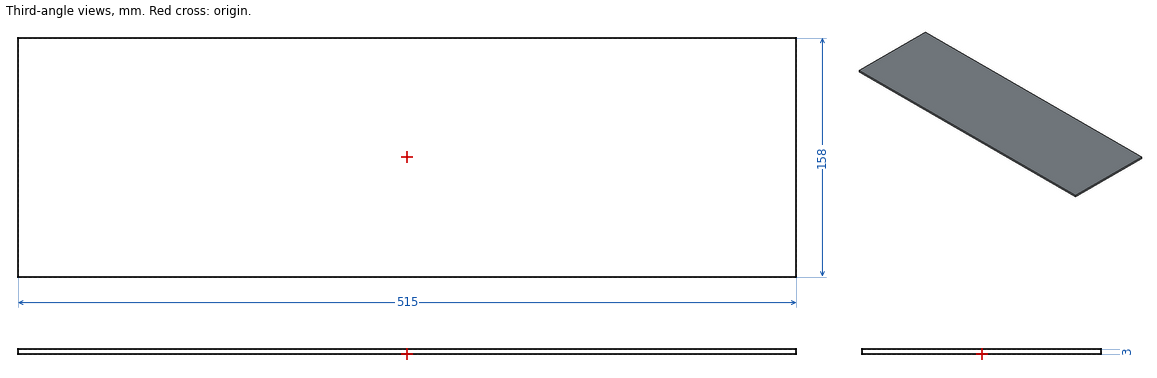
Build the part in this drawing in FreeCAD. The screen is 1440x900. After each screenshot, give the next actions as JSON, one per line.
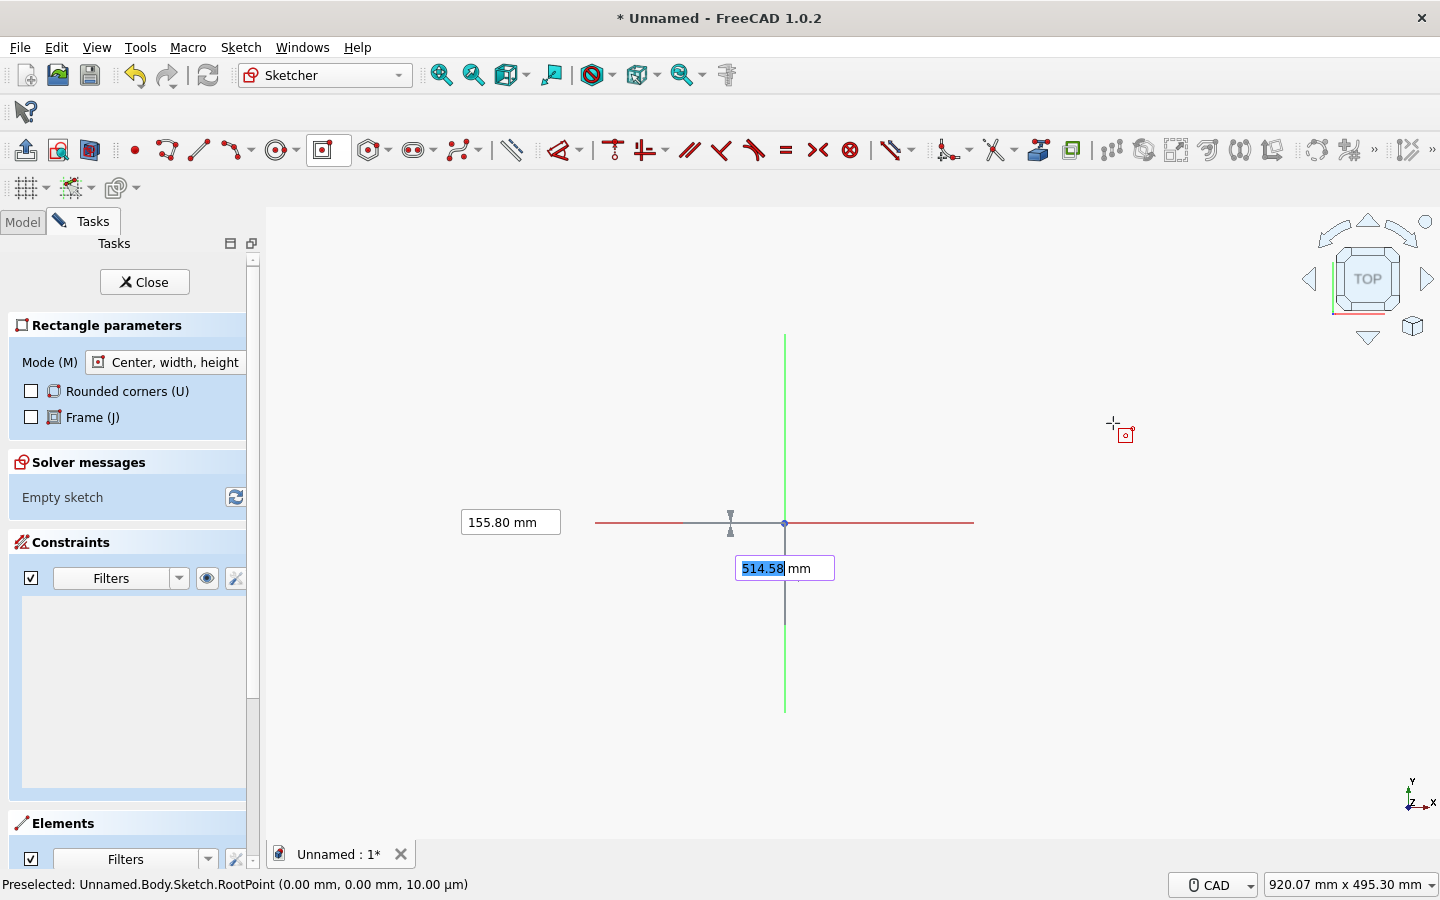
{"action": "type", "text": "515"}
{"action": "key", "text": "Tab"}
{"action": "type", "text": "158"}
{"action": "key", "text": "Return"}
{"action": "key", "text": "Escape"}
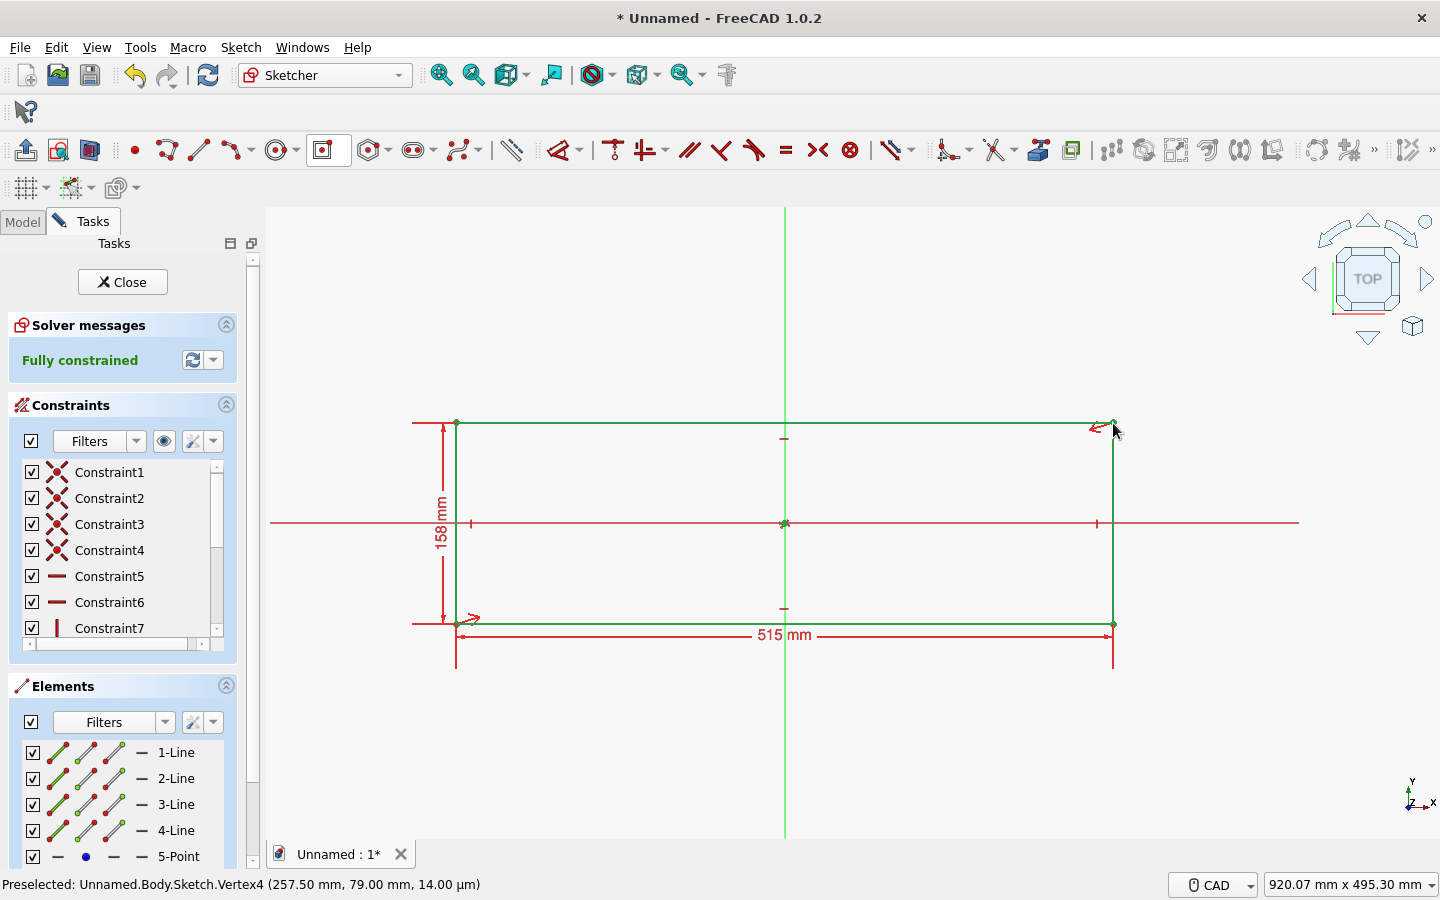
{"action": "left_click", "coordinate": [123, 282]}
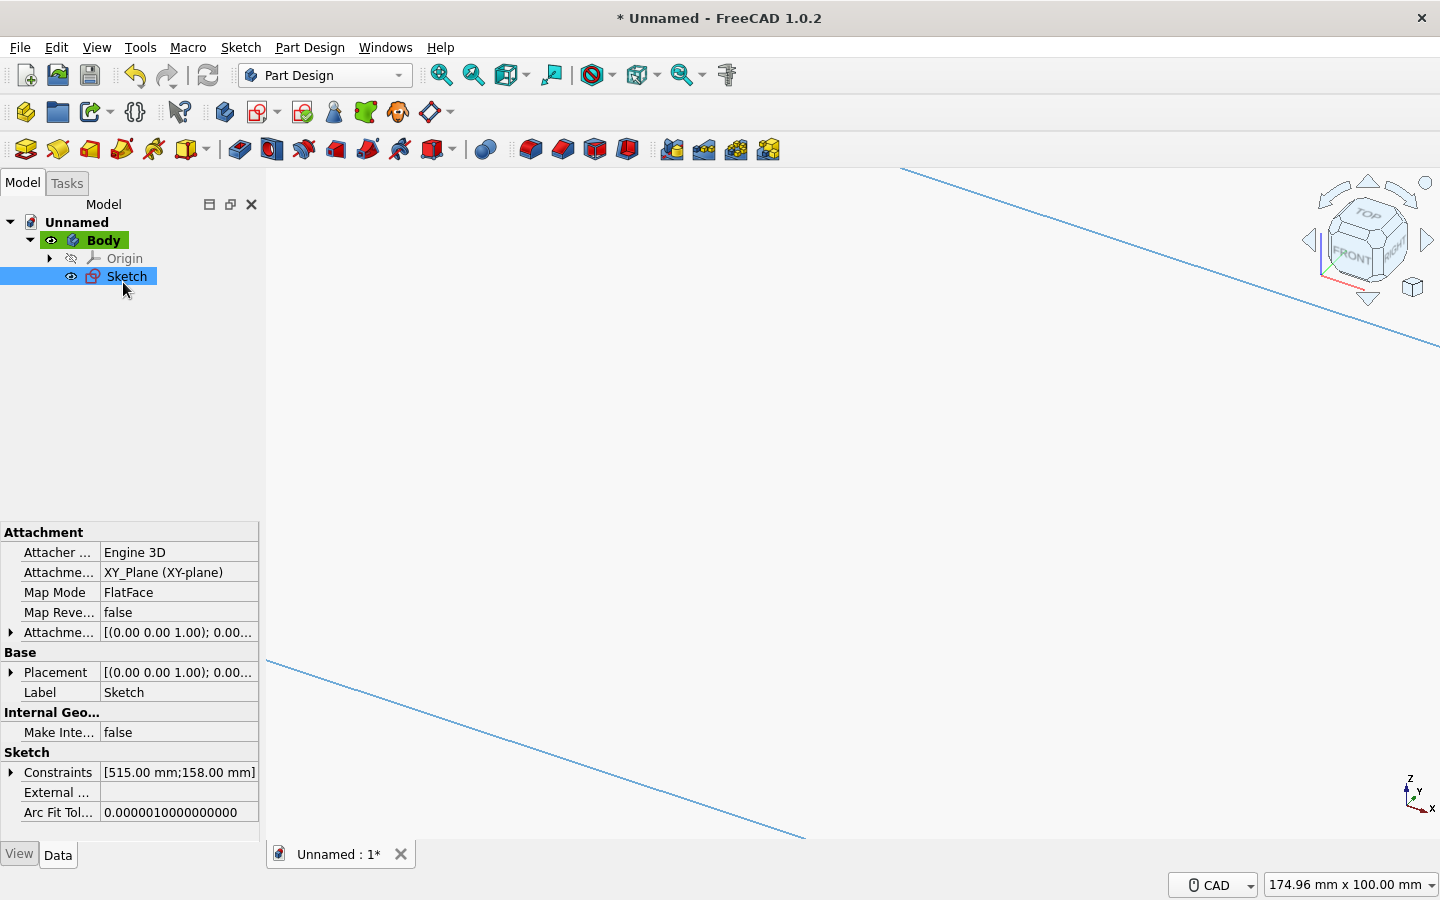
{"action": "left_click", "coordinate": [26, 150]}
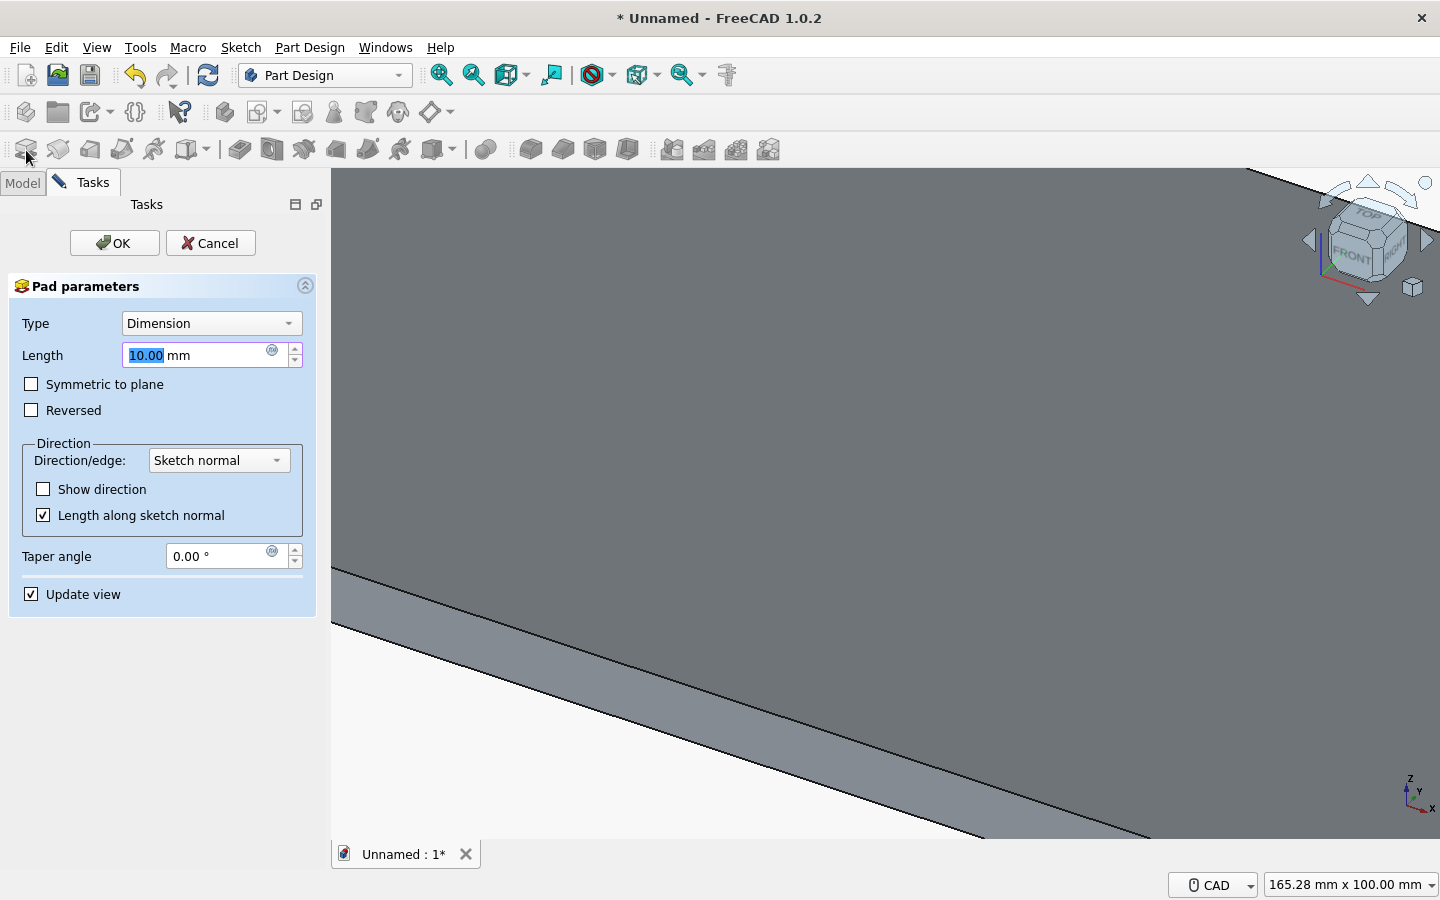
{"action": "type", "text": "3"}
{"action": "key", "text": "Tab"}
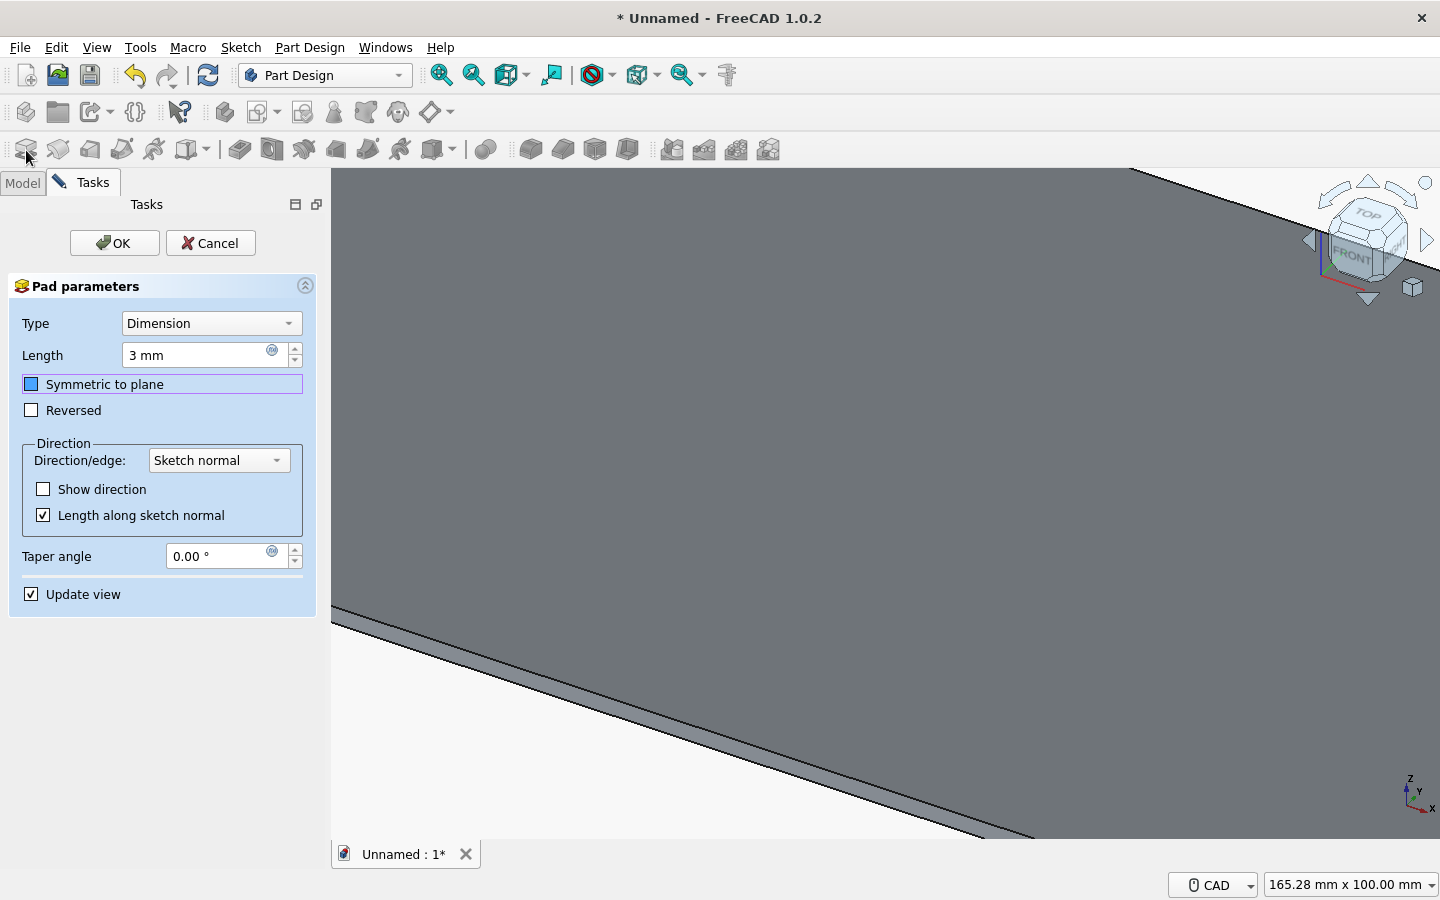
{"action": "left_click", "coordinate": [115, 243]}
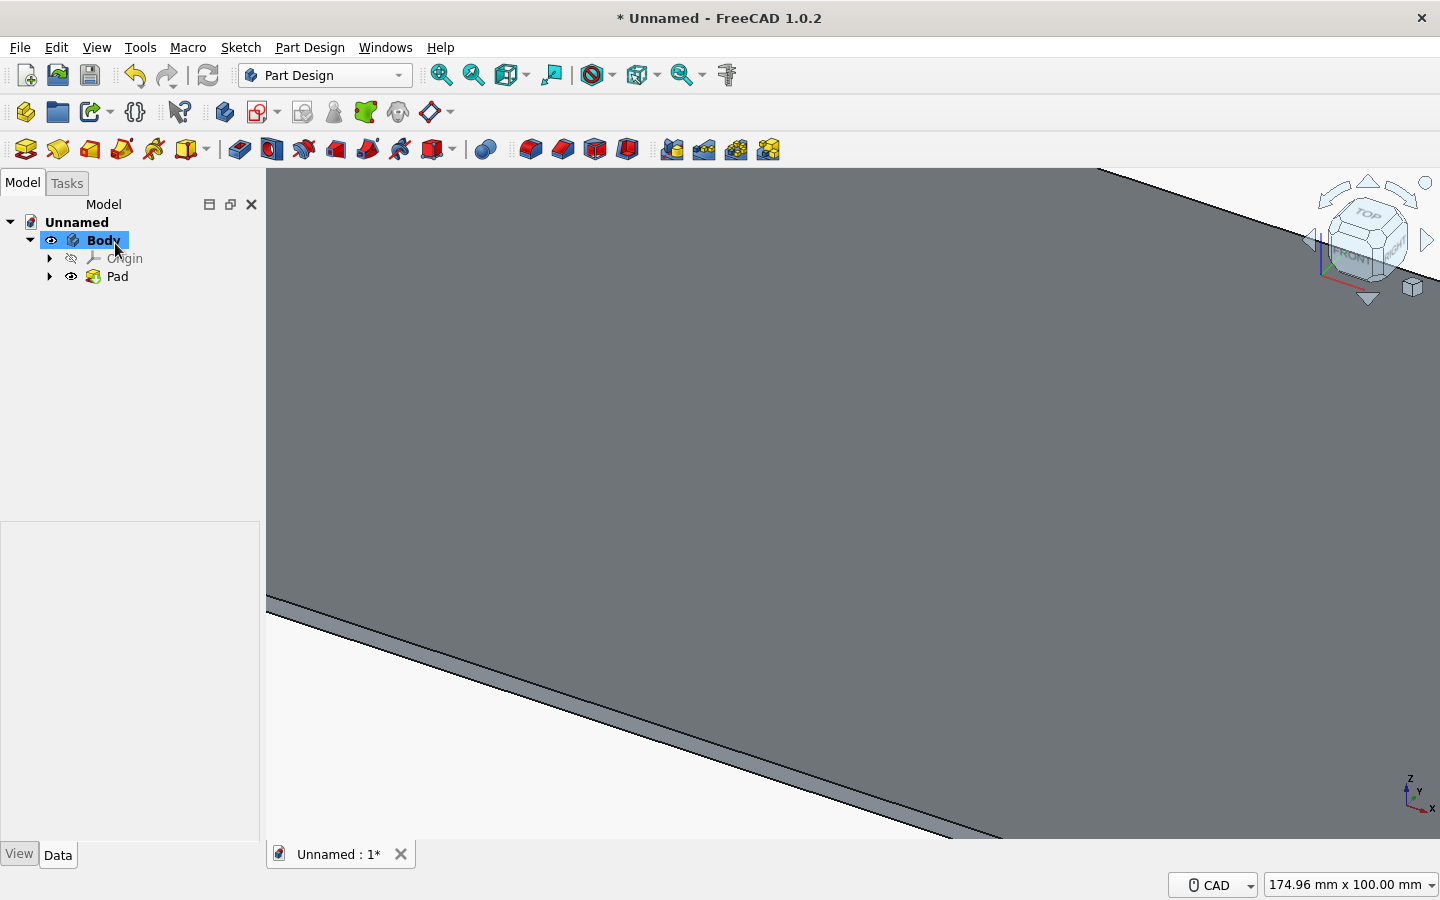
{"action": "key", "text": "0"}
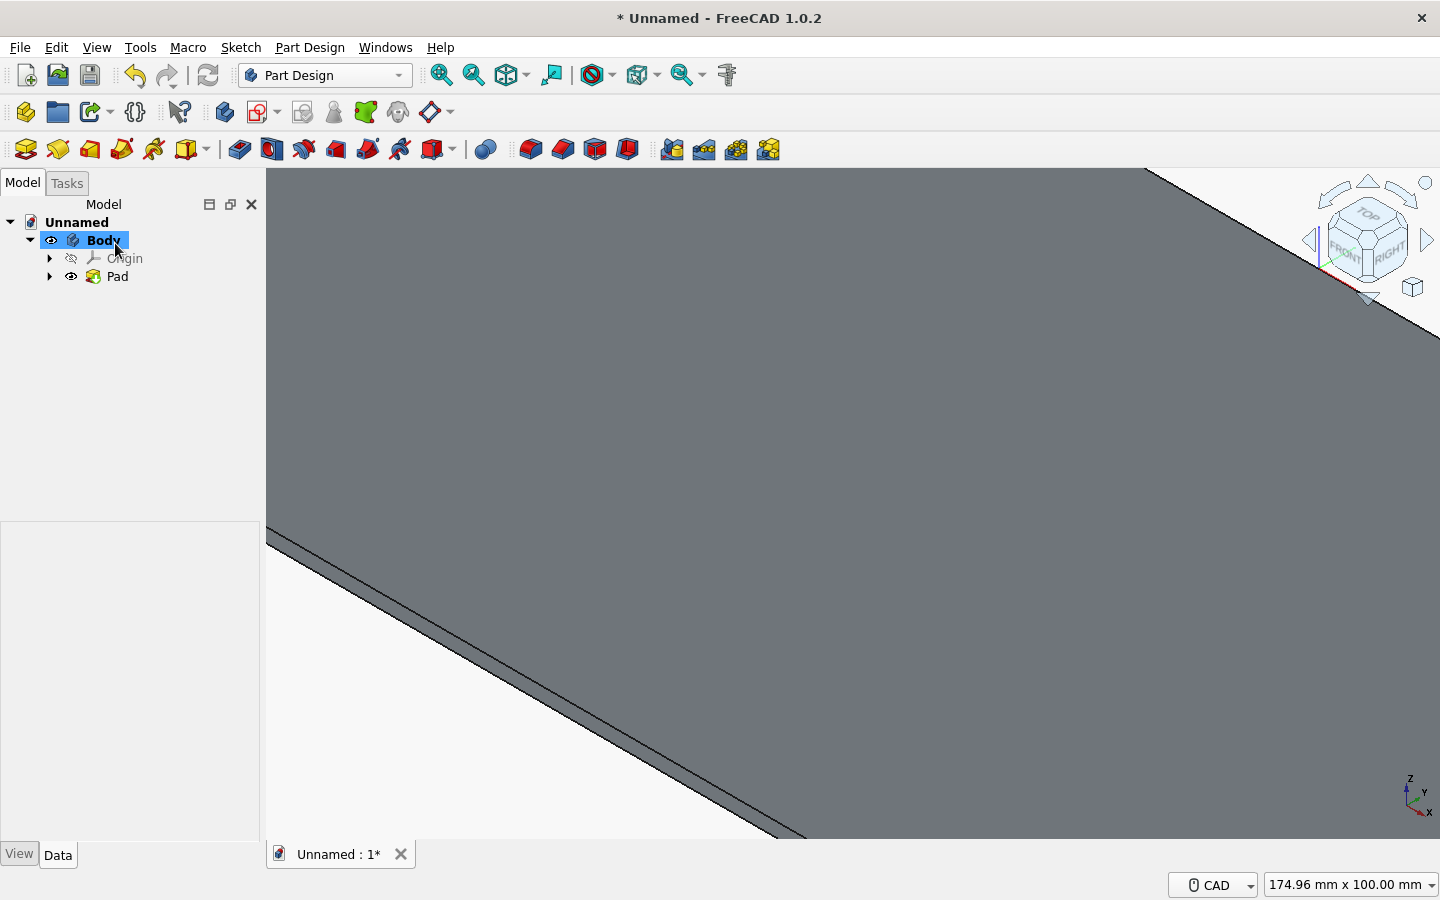
{"action": "left_click", "coordinate": [442, 76]}